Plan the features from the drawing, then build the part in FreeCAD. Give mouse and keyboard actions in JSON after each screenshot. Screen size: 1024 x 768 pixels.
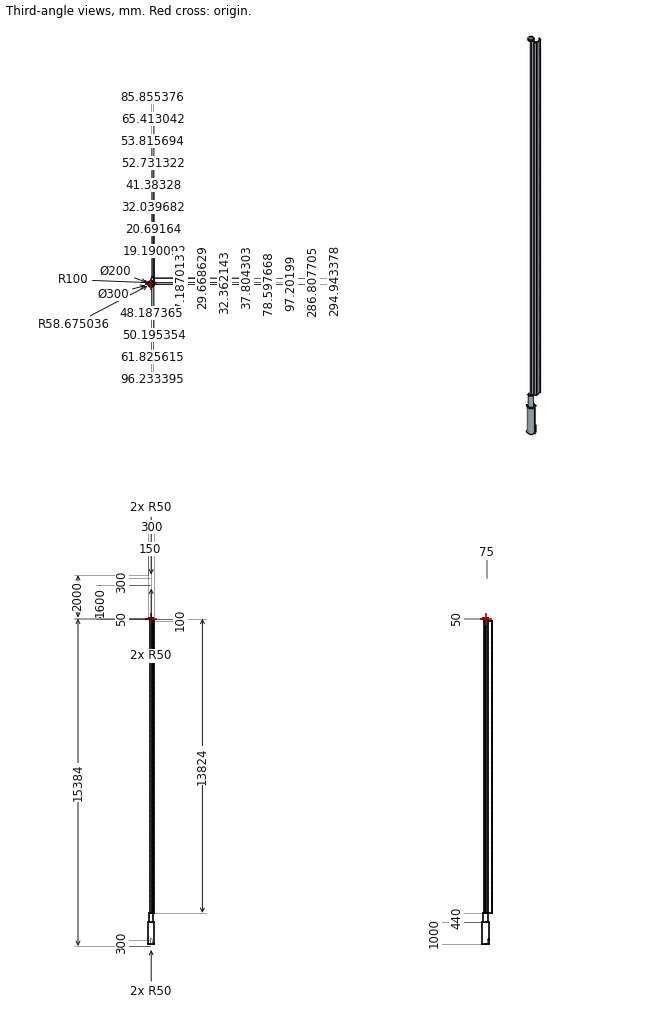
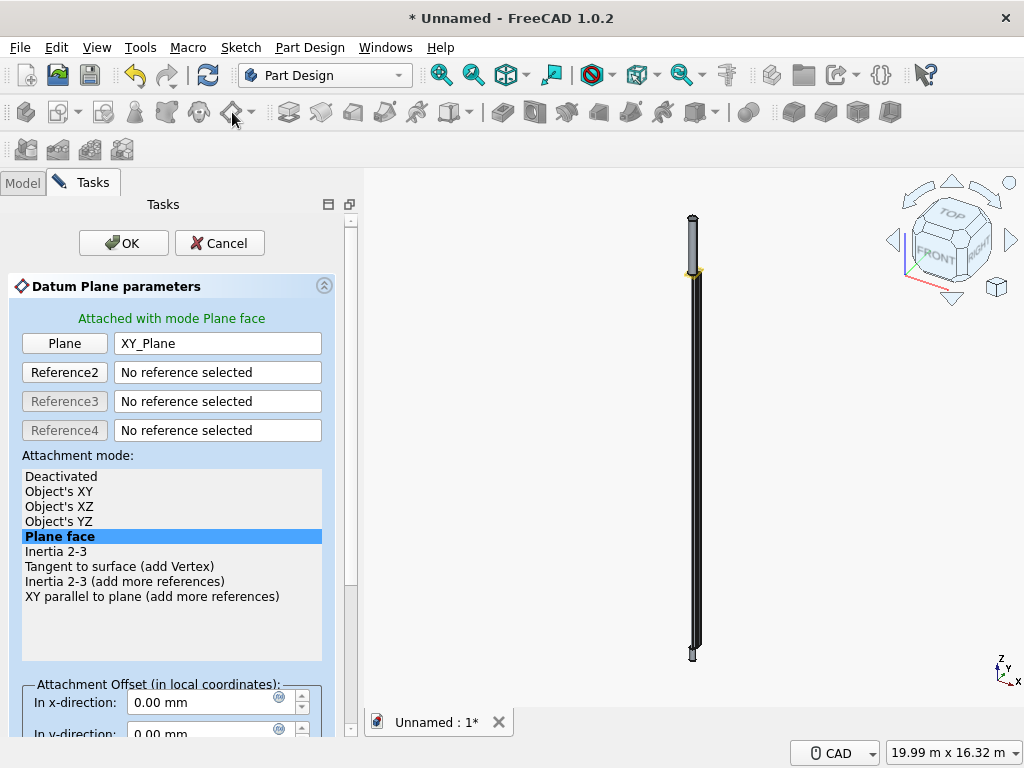
{"action": "scroll", "coordinate": [351, 475], "scroll_direction": "down", "scroll_amount": 2}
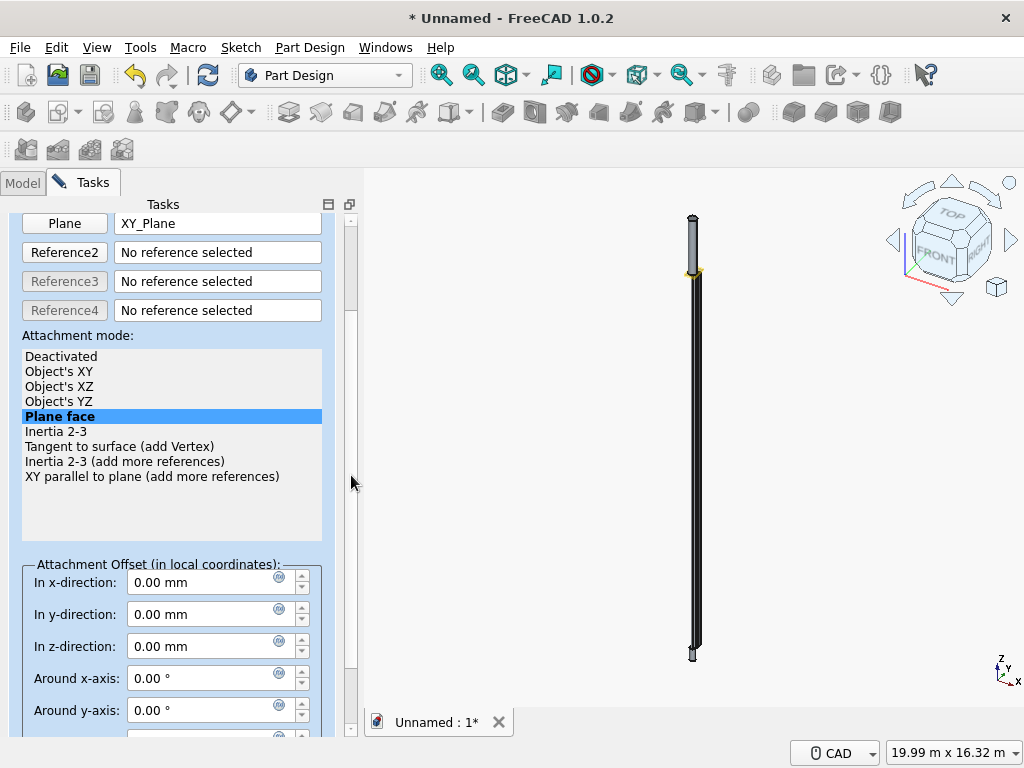
{"action": "triple_click", "coordinate": [210, 646]}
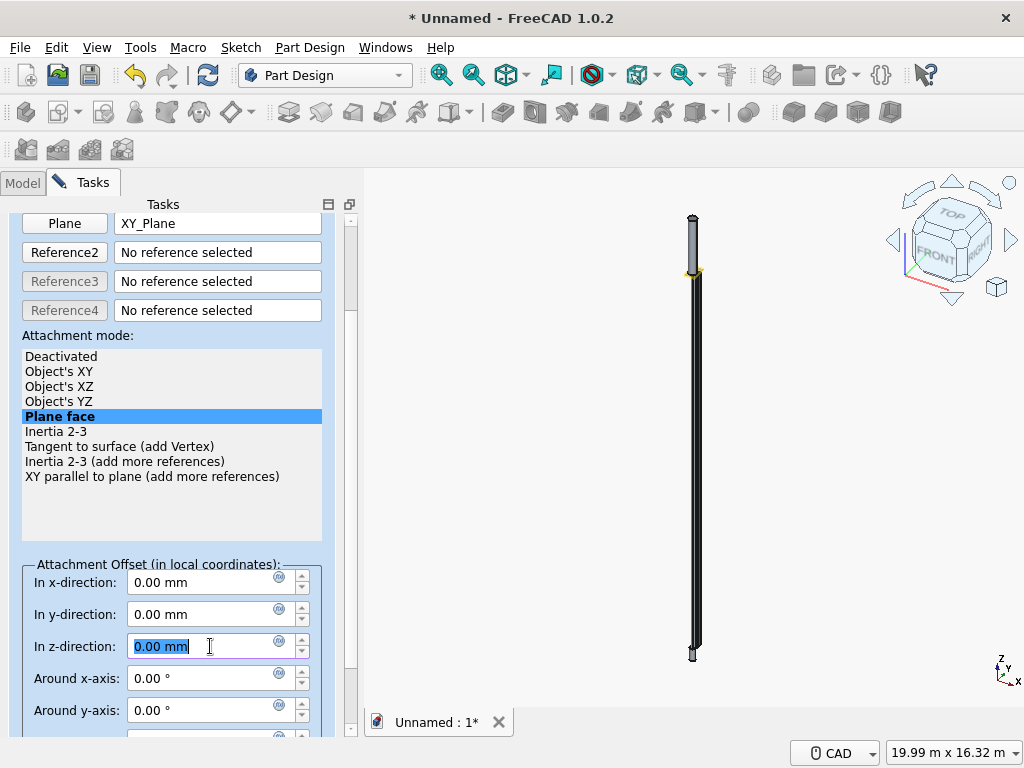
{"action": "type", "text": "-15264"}
{"action": "key", "text": "Tab"}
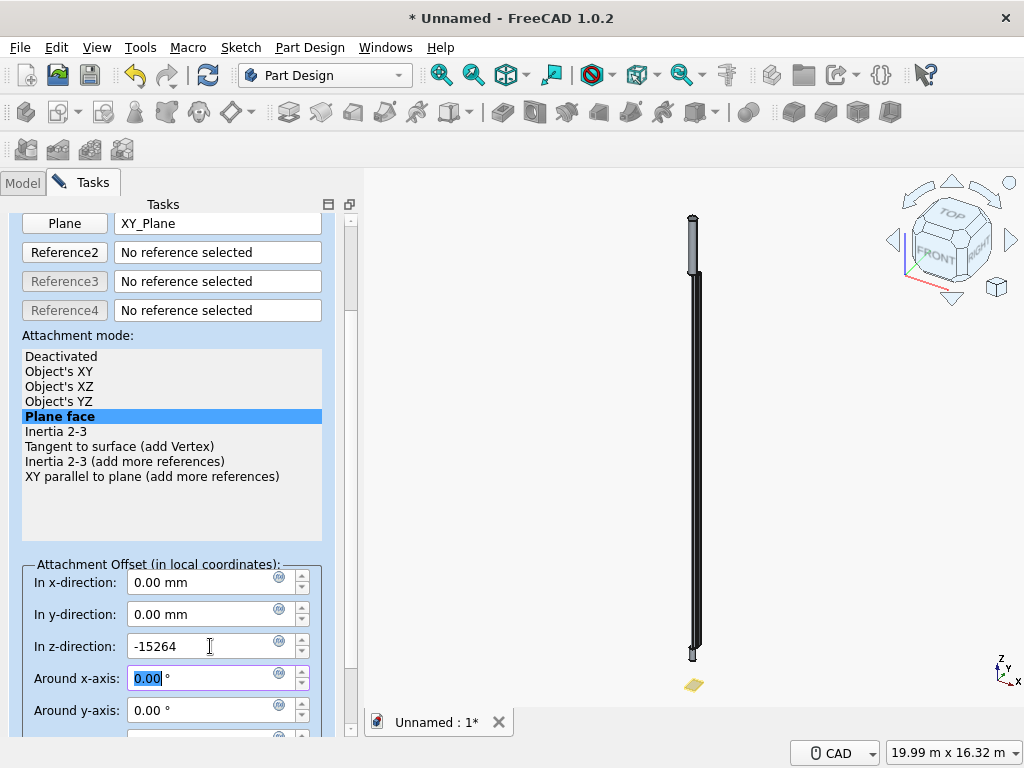
{"action": "scroll", "coordinate": [351, 475], "scroll_direction": "up", "scroll_amount": 3}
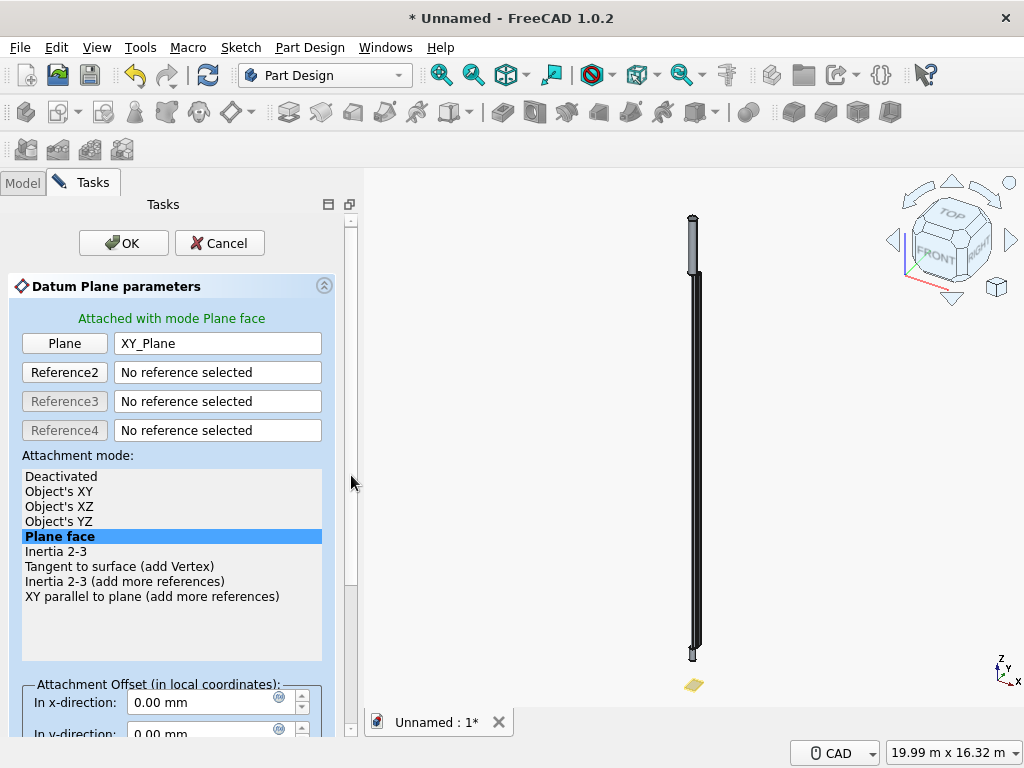
{"action": "left_click", "coordinate": [124, 243]}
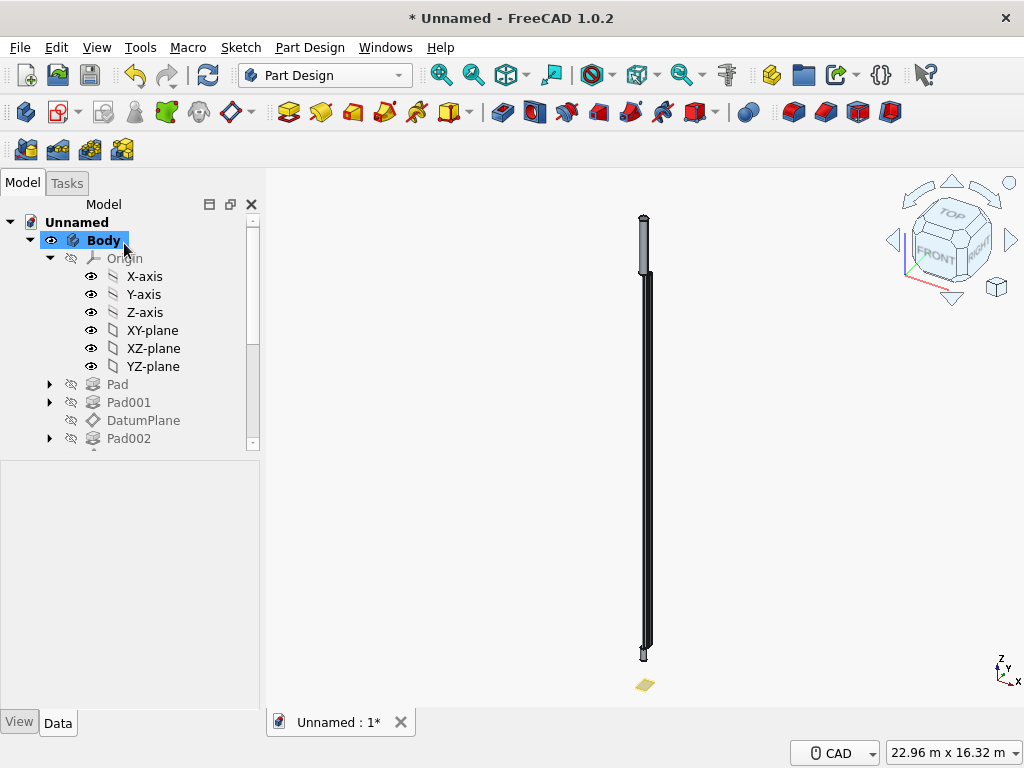
{"action": "scroll", "coordinate": [100, 326], "scroll_direction": "down", "scroll_amount": 3}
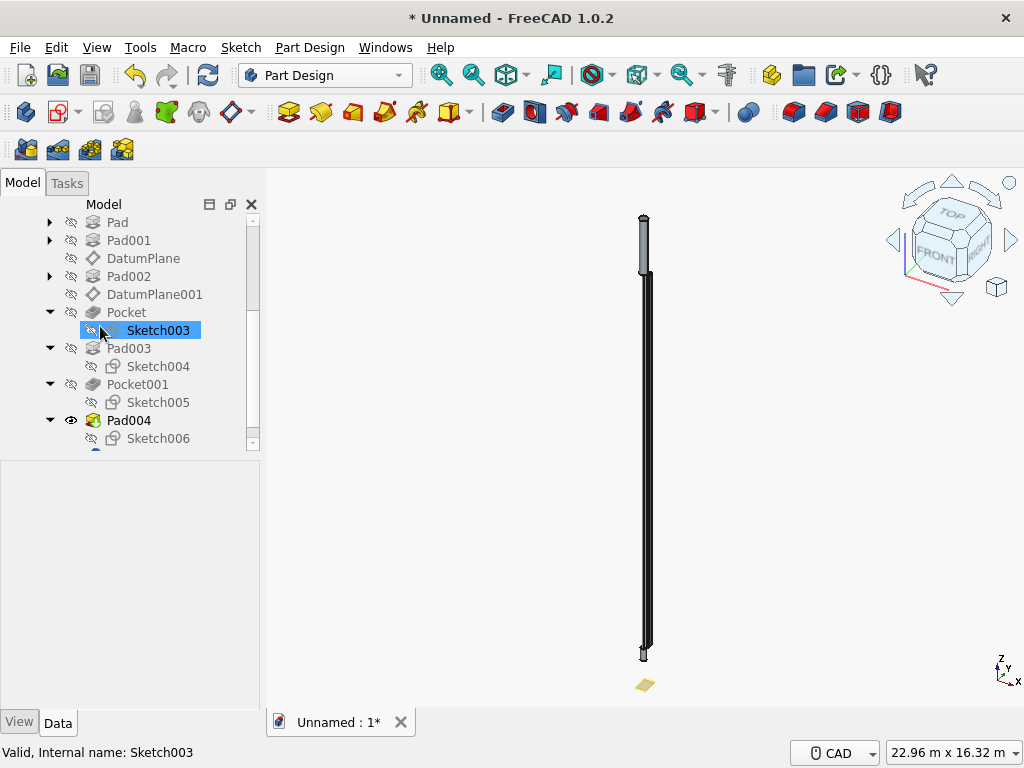
{"action": "scroll", "coordinate": [140, 326], "scroll_direction": "up", "scroll_amount": 15}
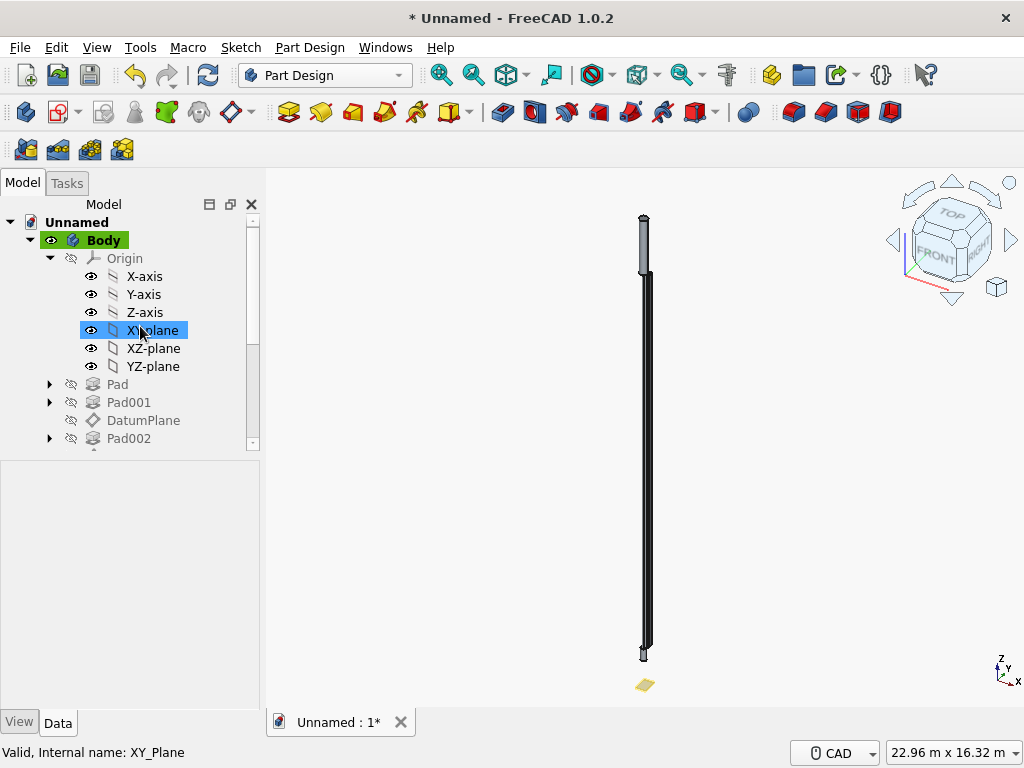
{"action": "scroll", "coordinate": [100, 326], "scroll_direction": "down", "scroll_amount": 6}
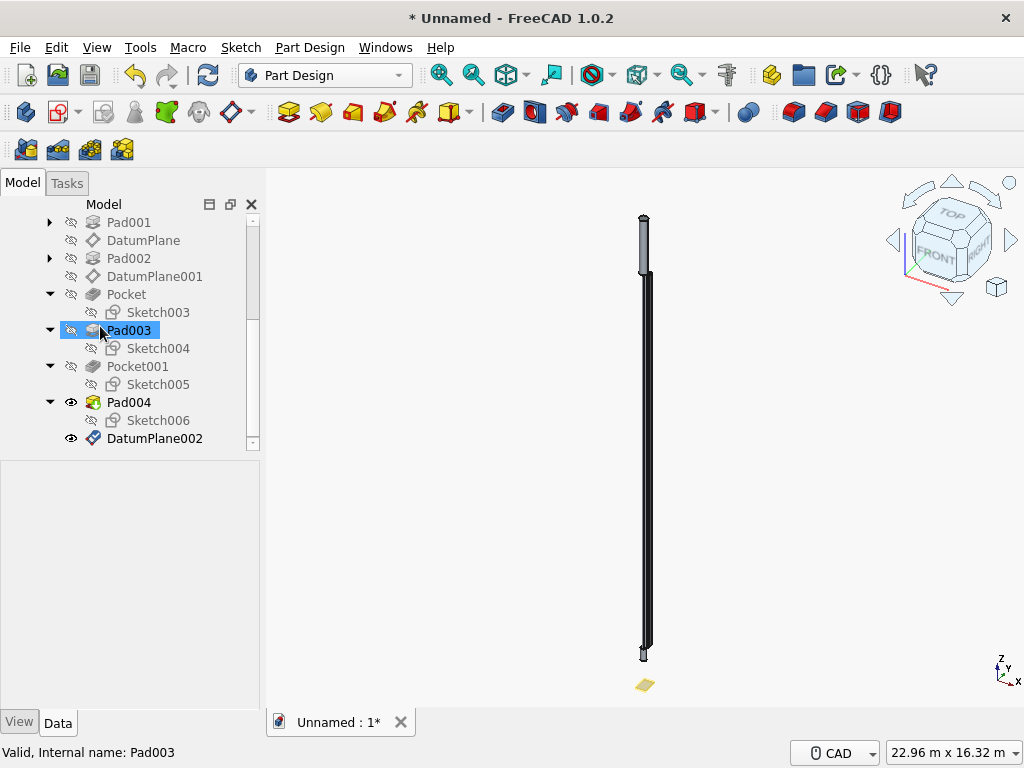
{"action": "left_click", "coordinate": [116, 438]}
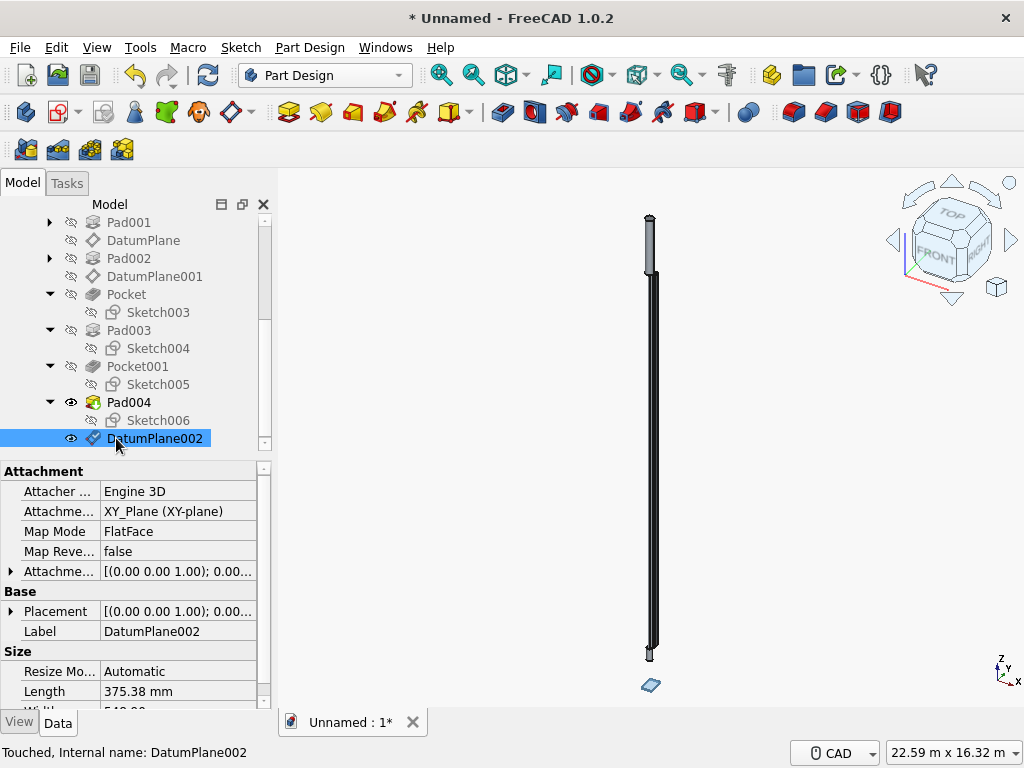
{"action": "left_click", "coordinate": [58, 112]}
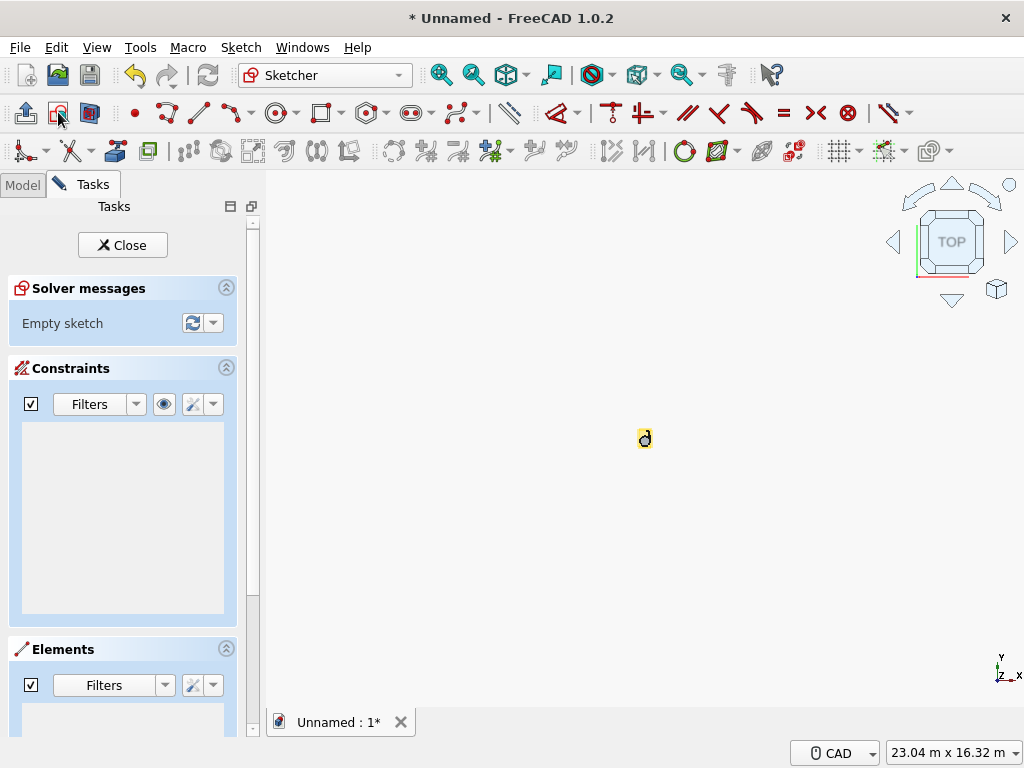
{"action": "left_click", "coordinate": [90, 114]}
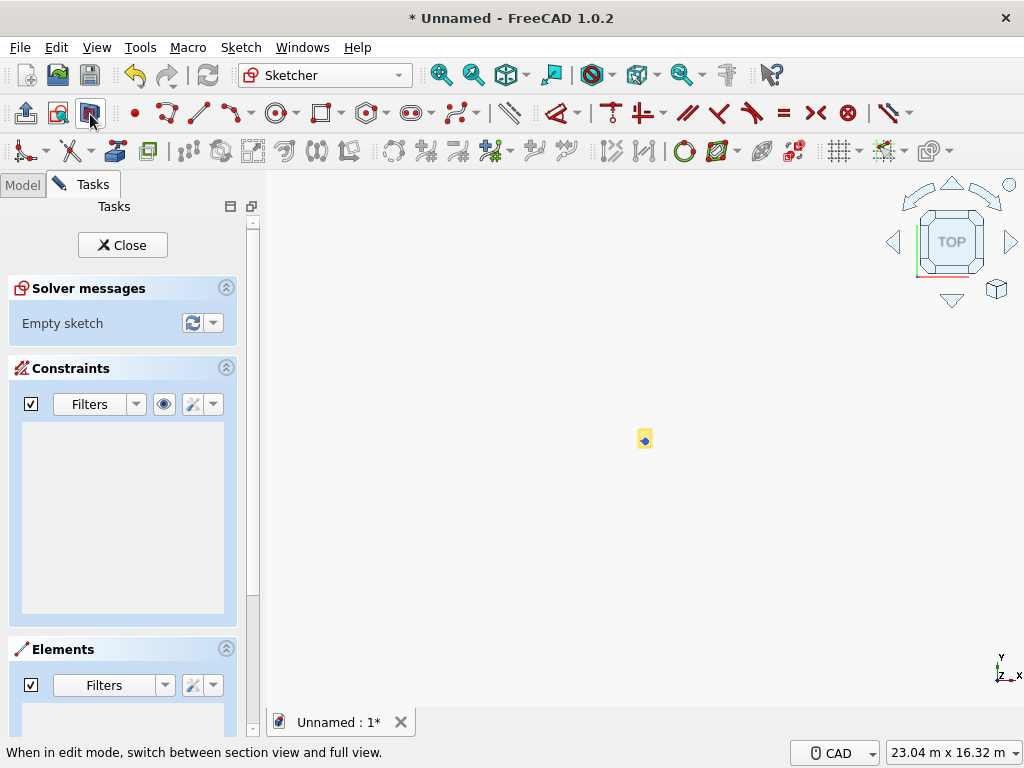
{"action": "scroll", "coordinate": [649, 442], "scroll_direction": "up", "scroll_amount": 15}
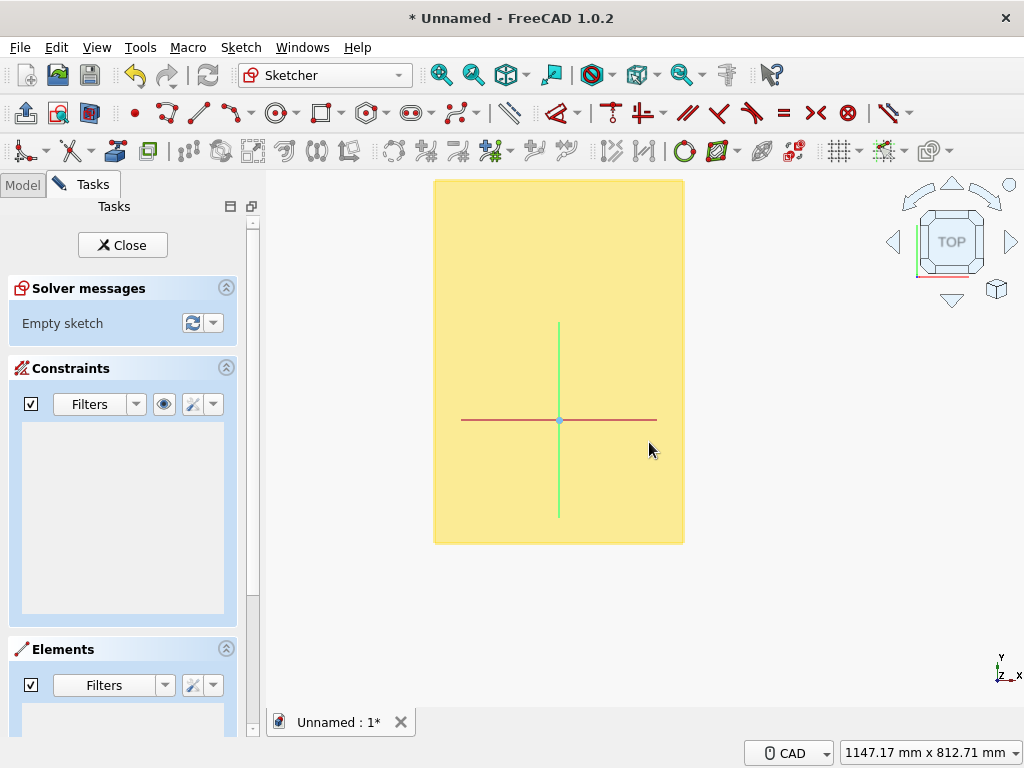
{"action": "scroll", "coordinate": [538, 398], "scroll_direction": "up", "scroll_amount": 3}